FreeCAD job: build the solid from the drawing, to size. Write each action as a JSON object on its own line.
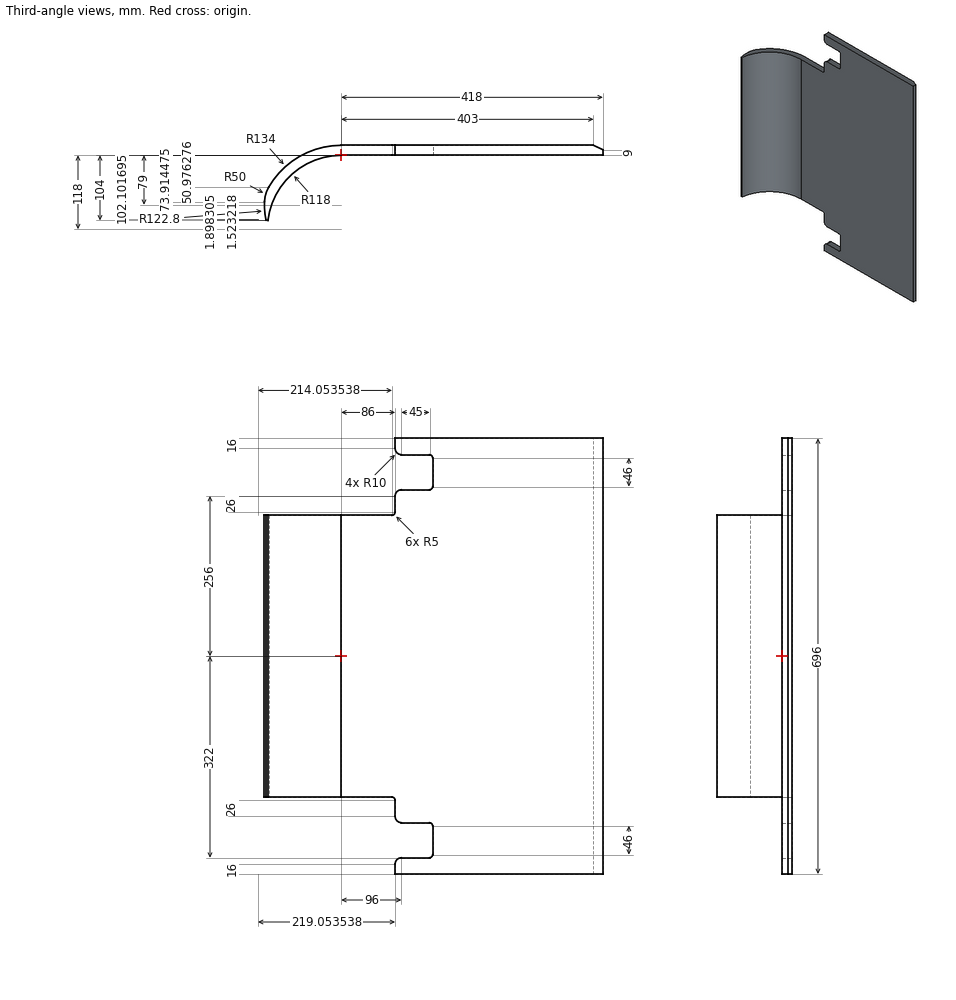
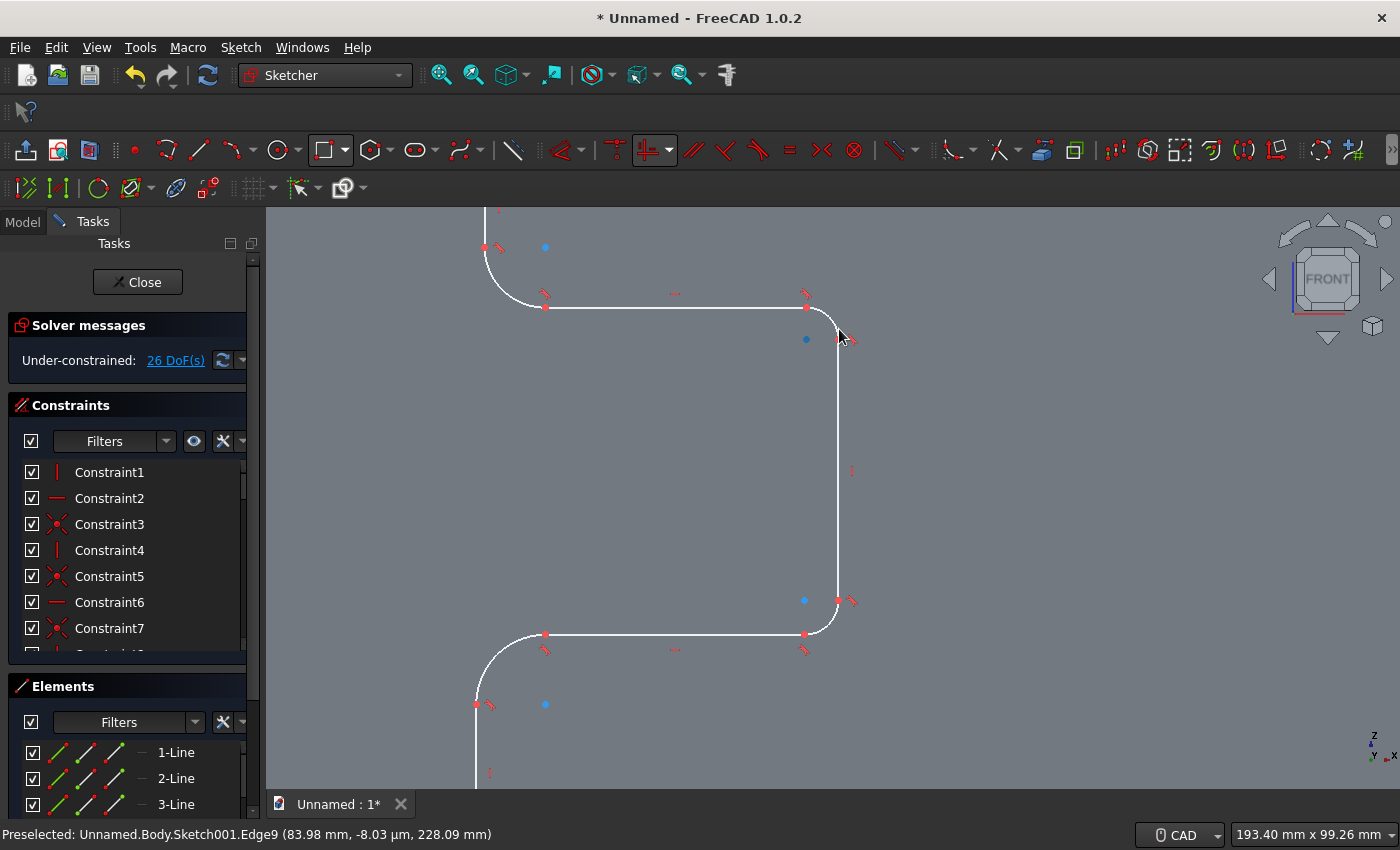
{"action": "left_click", "coordinate": [835, 325]}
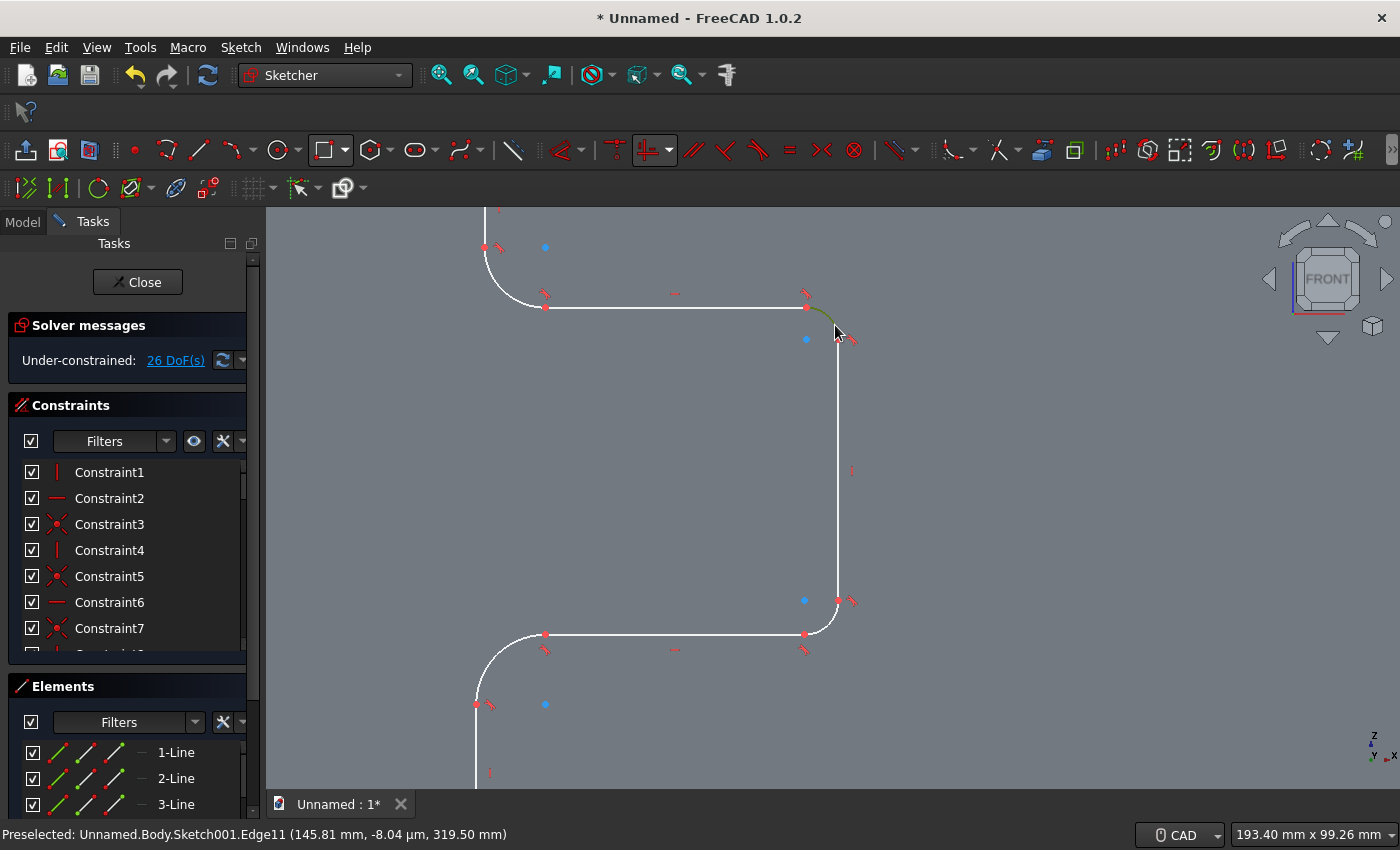
{"action": "left_click", "coordinate": [820, 631]}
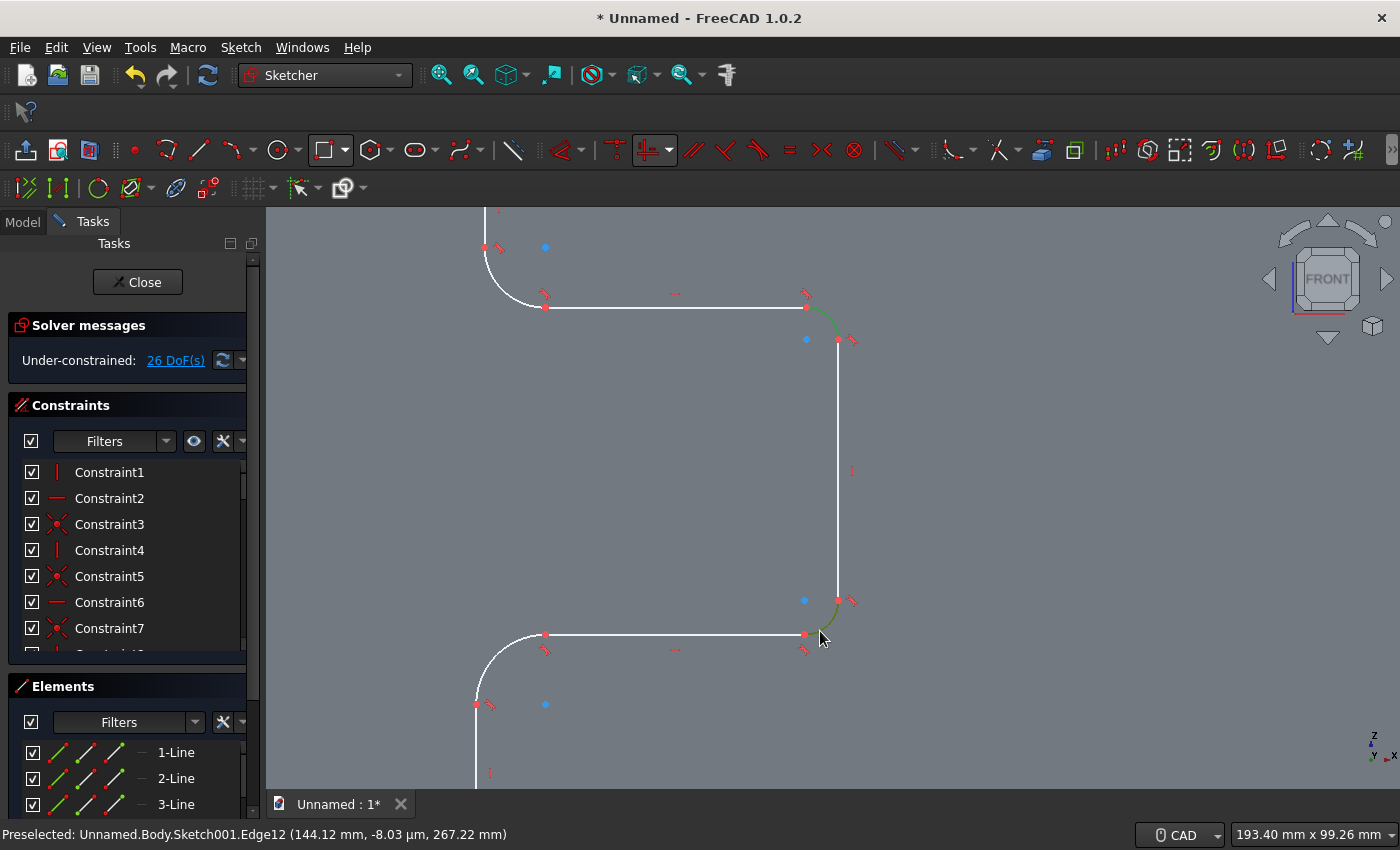
{"action": "scroll", "coordinate": [839, 329], "scroll_direction": "down", "scroll_amount": 12}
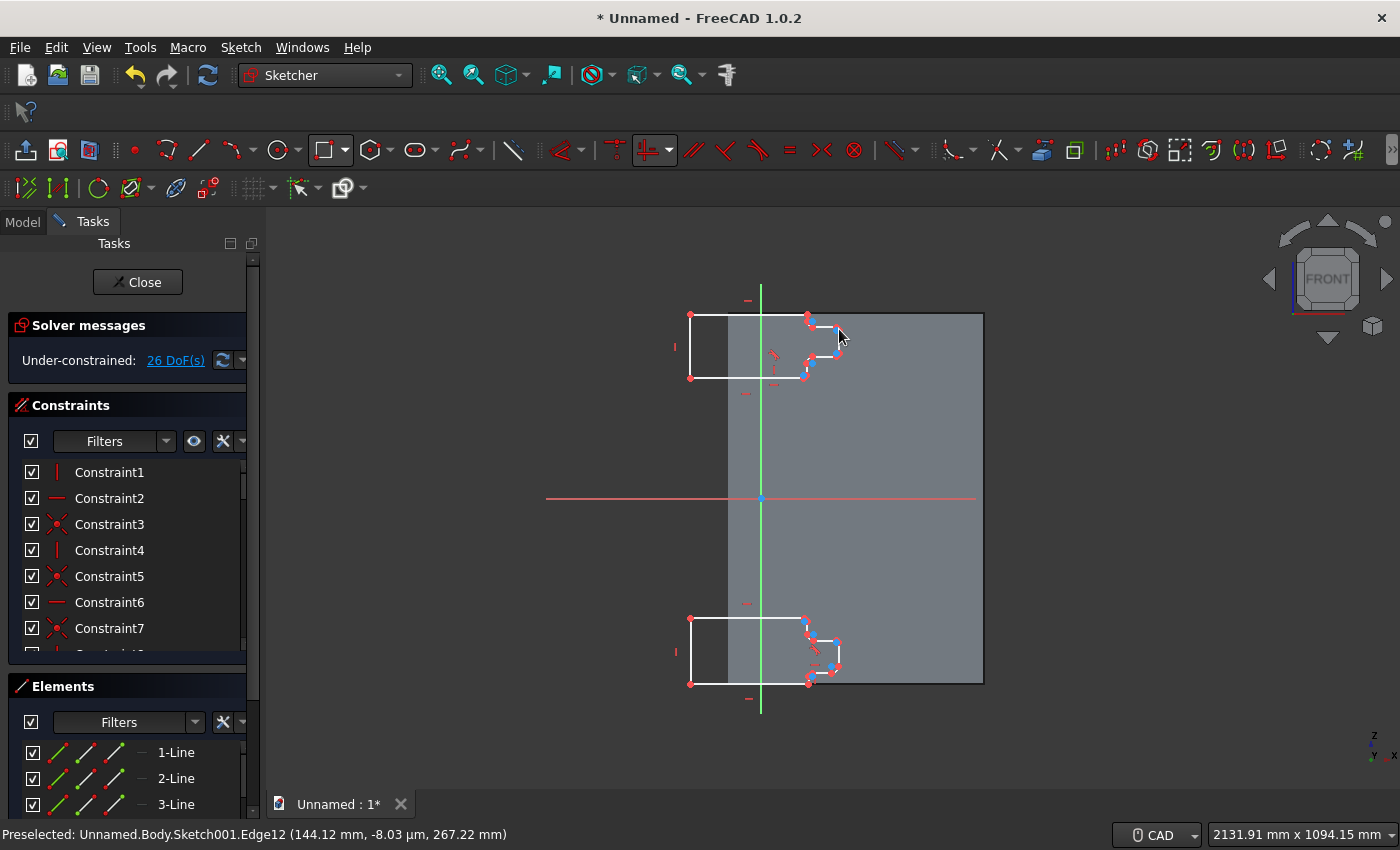
{"action": "scroll", "coordinate": [807, 620], "scroll_direction": "up", "scroll_amount": 12}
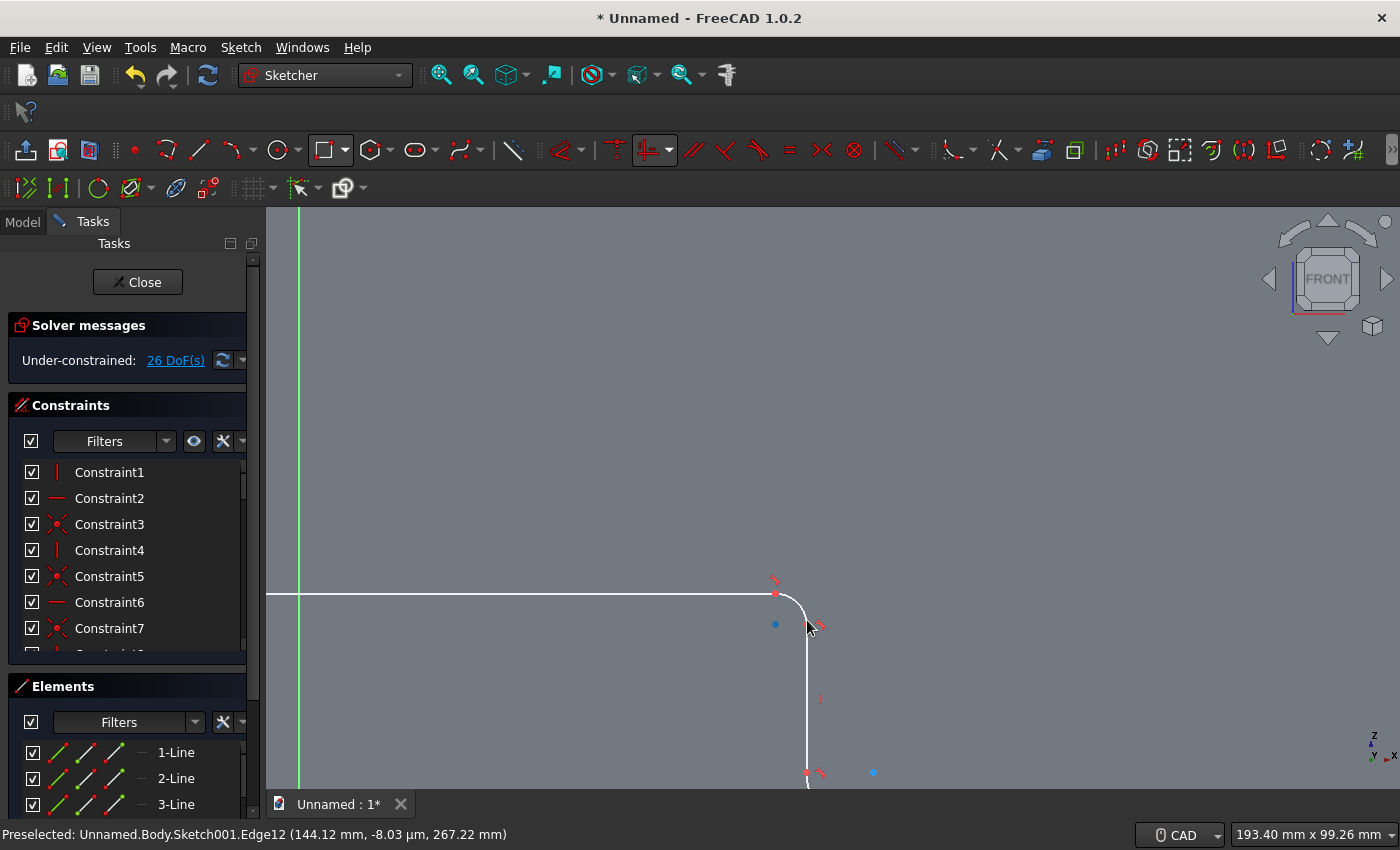
{"action": "left_click", "coordinate": [803, 611]}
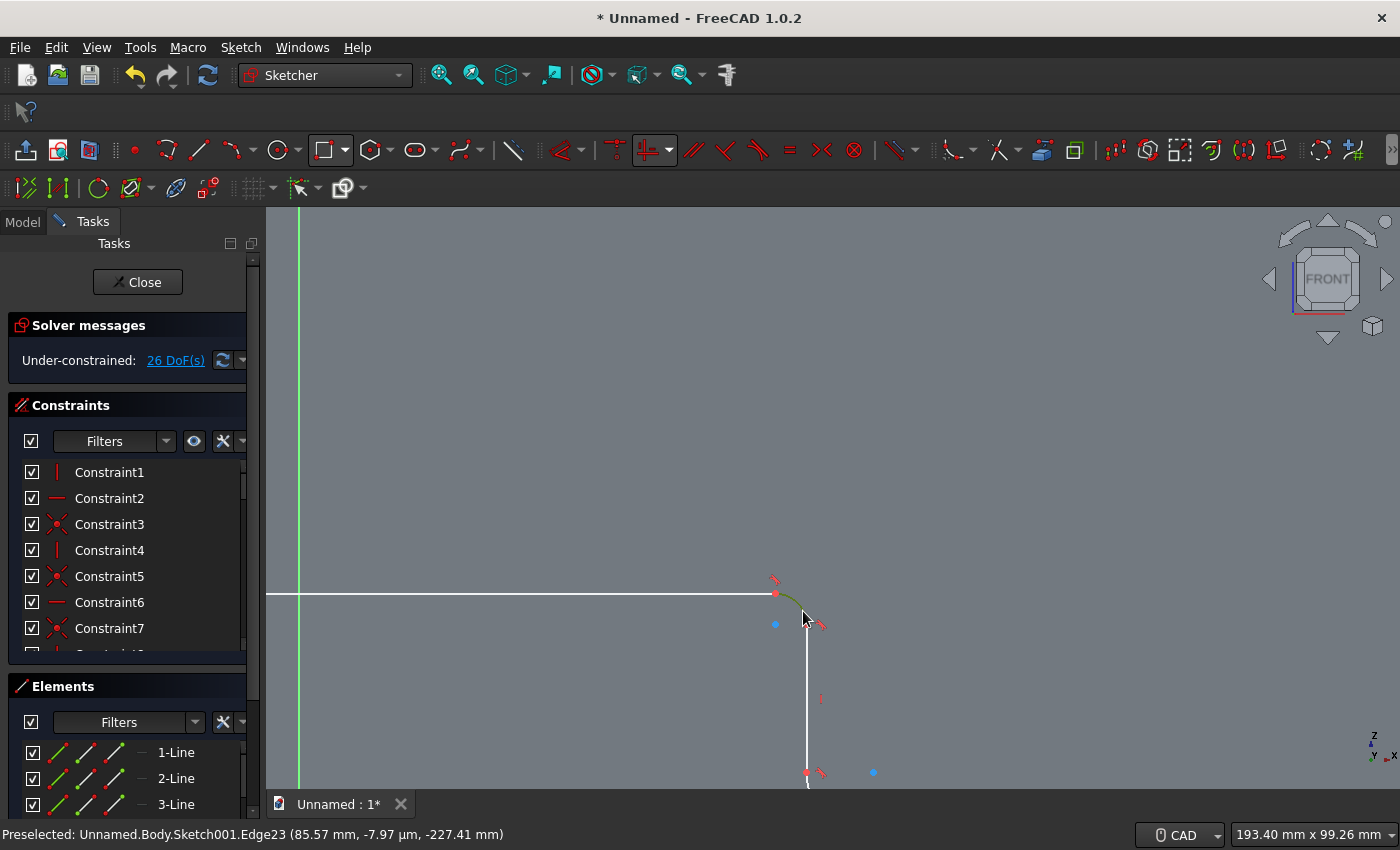
{"action": "scroll", "coordinate": [807, 620], "scroll_direction": "down", "scroll_amount": 12}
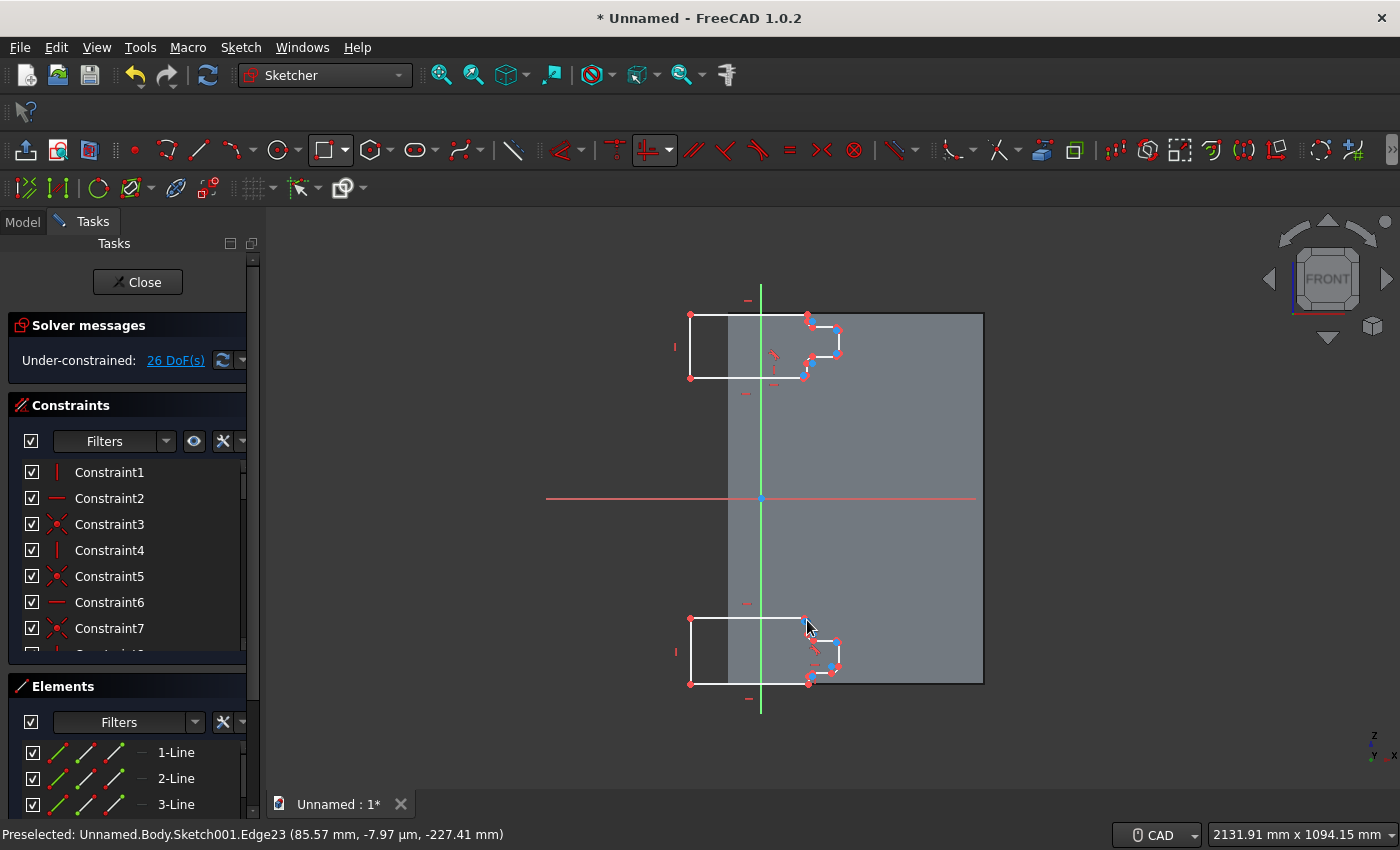
{"action": "scroll", "coordinate": [838, 642], "scroll_direction": "up", "scroll_amount": 13}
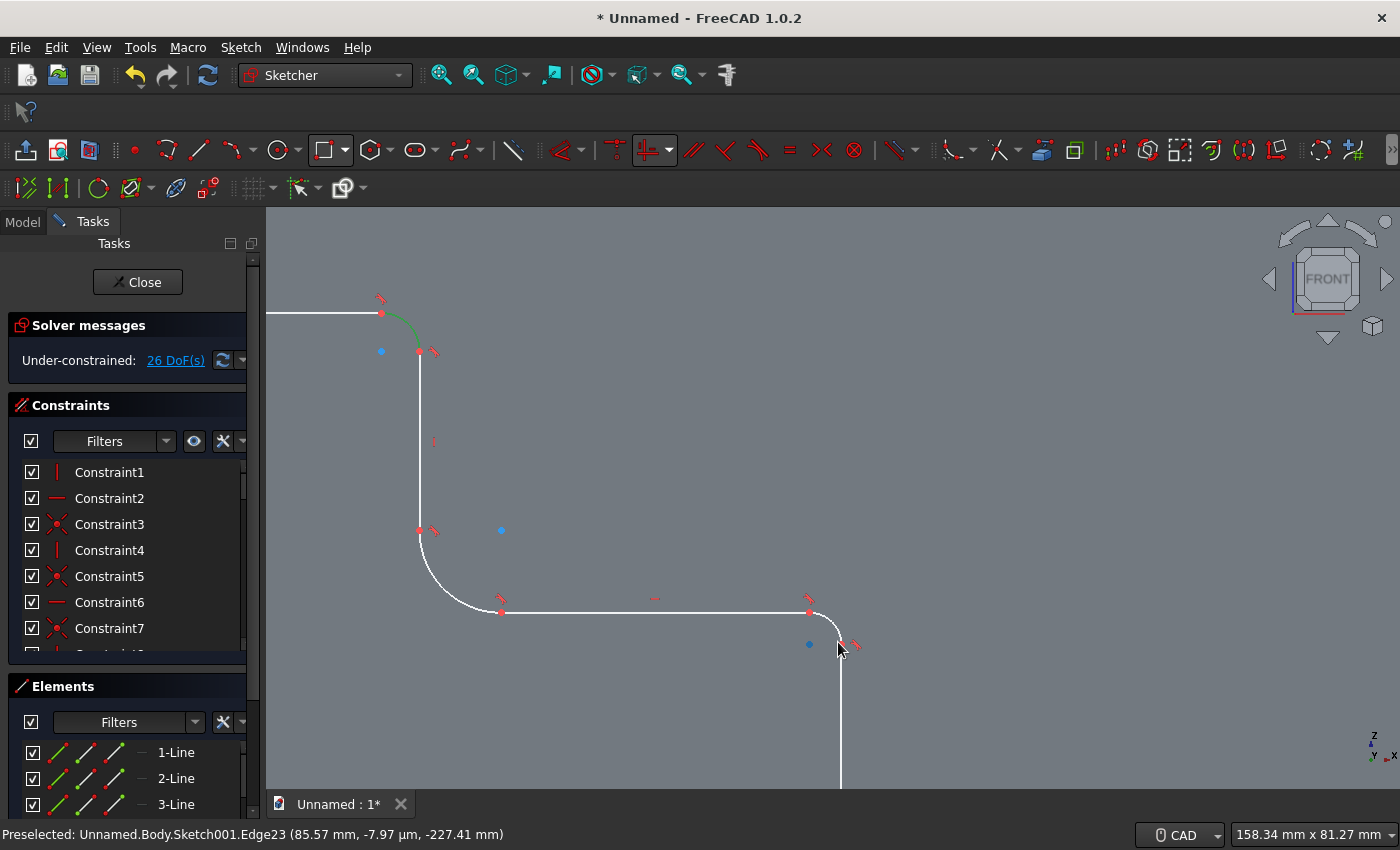
{"action": "left_click", "coordinate": [838, 630]}